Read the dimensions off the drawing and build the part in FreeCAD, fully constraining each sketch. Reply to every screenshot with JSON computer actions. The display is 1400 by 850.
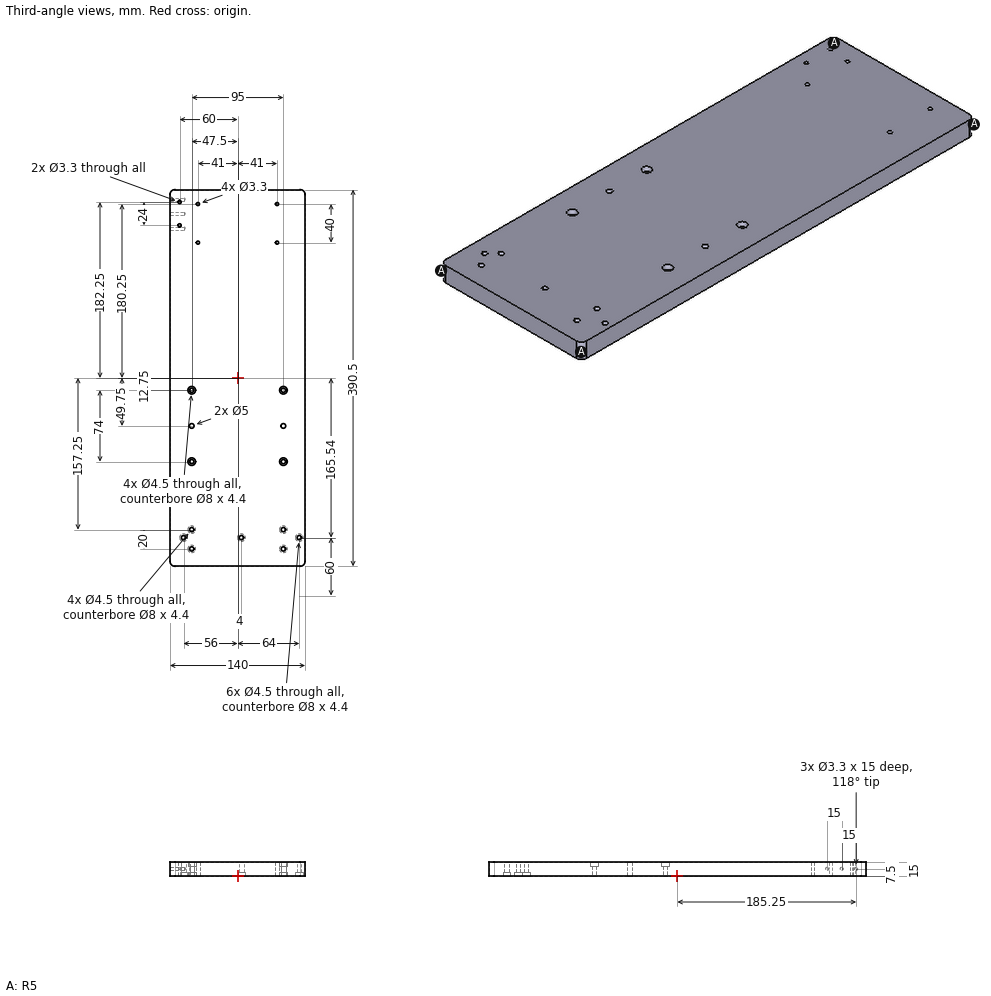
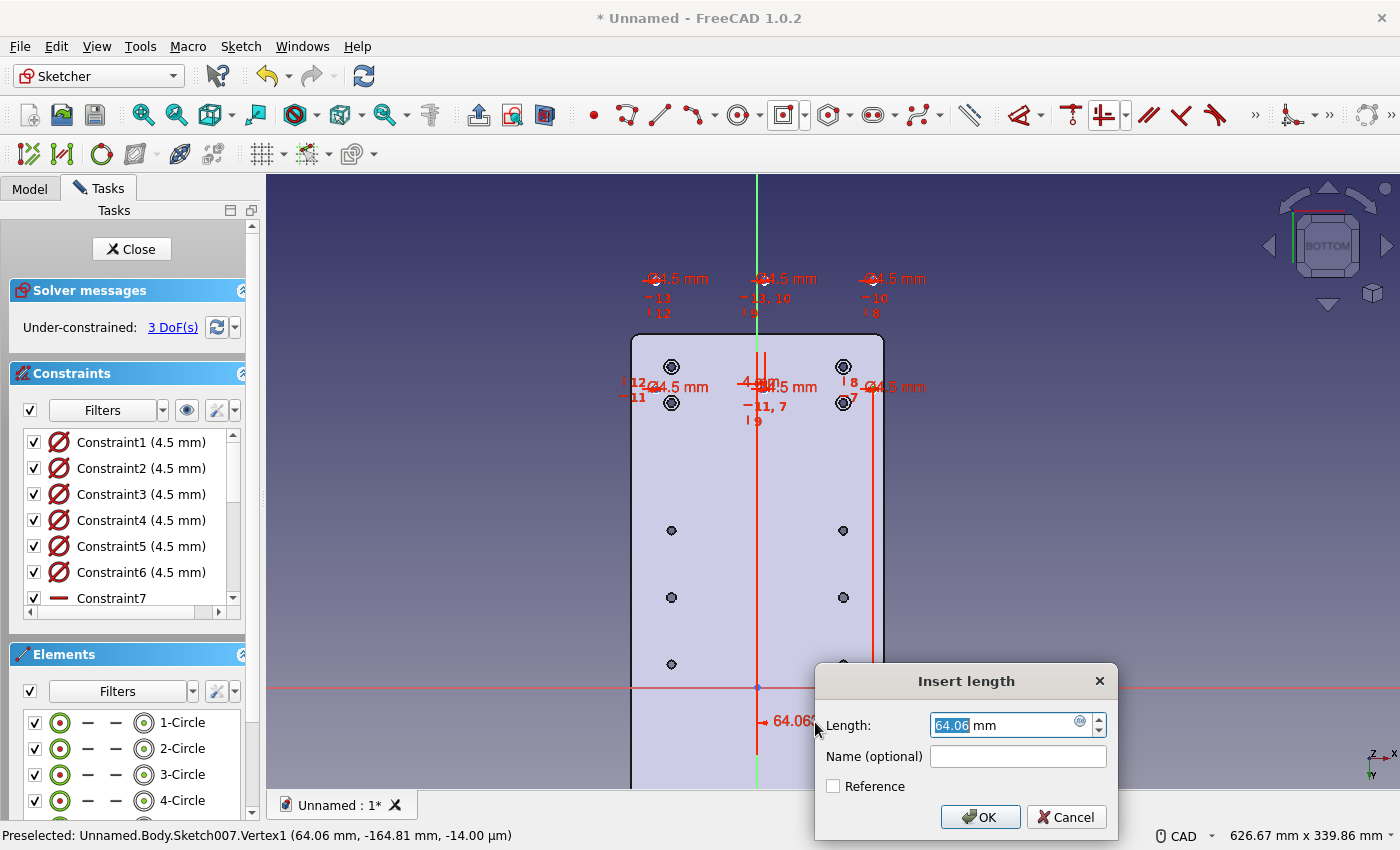
{"action": "type", "text": "64"}
{"action": "key", "text": "Return"}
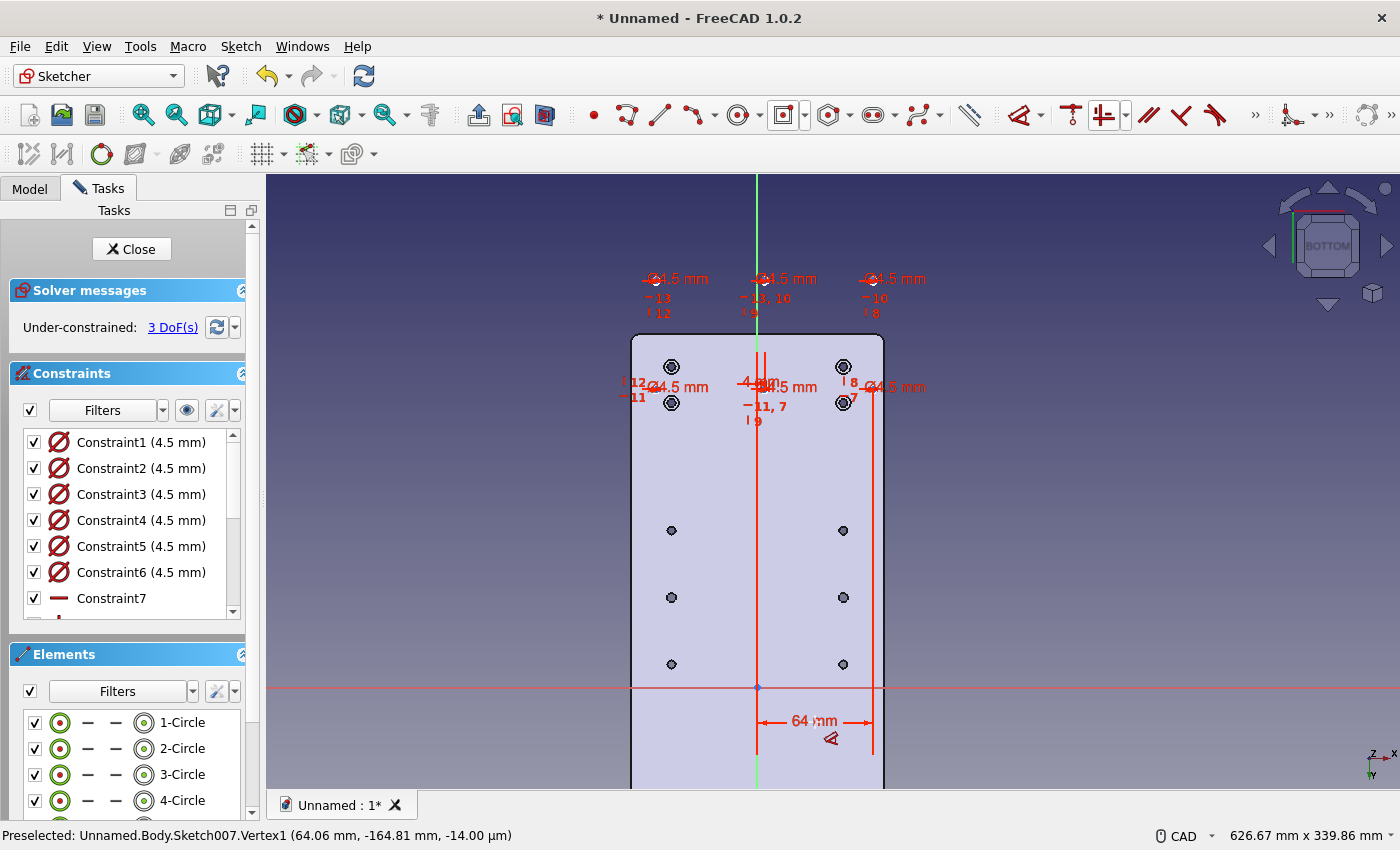
{"action": "left_click", "coordinate": [656, 389]}
{"action": "left_click", "coordinate": [707, 722]}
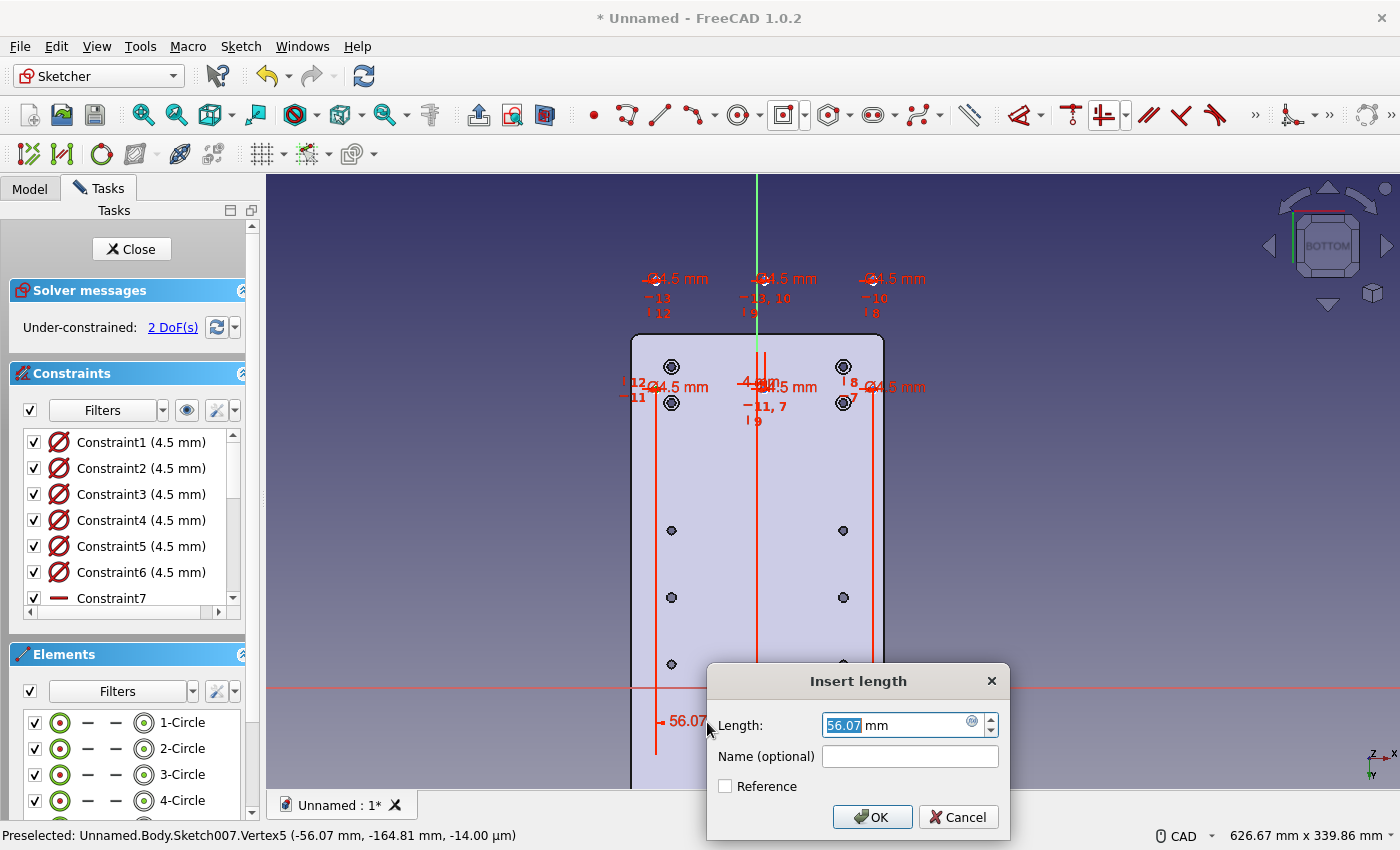
{"action": "type", "text": "56"}
{"action": "key", "text": "Return"}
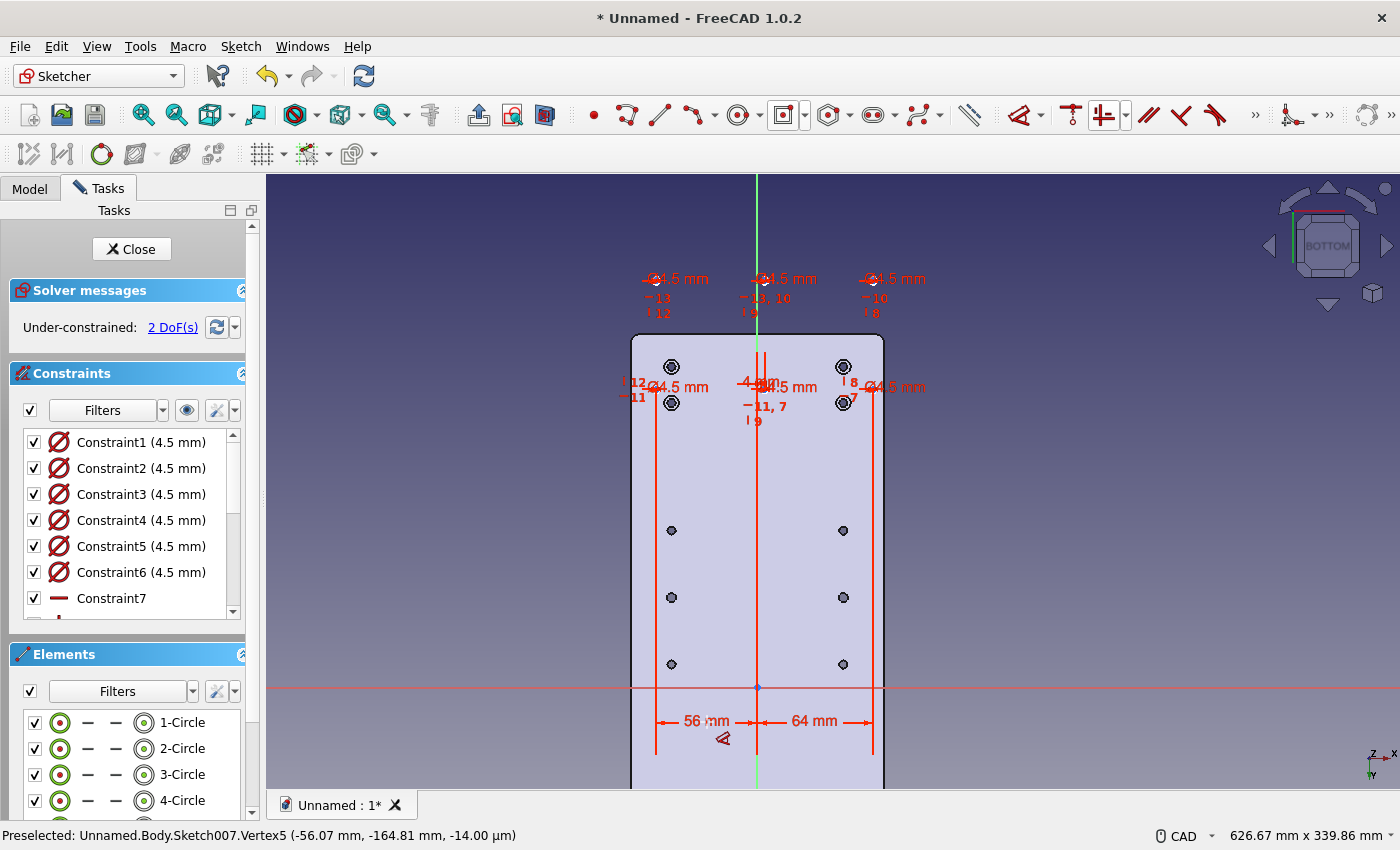
{"action": "left_click", "coordinate": [873, 389]}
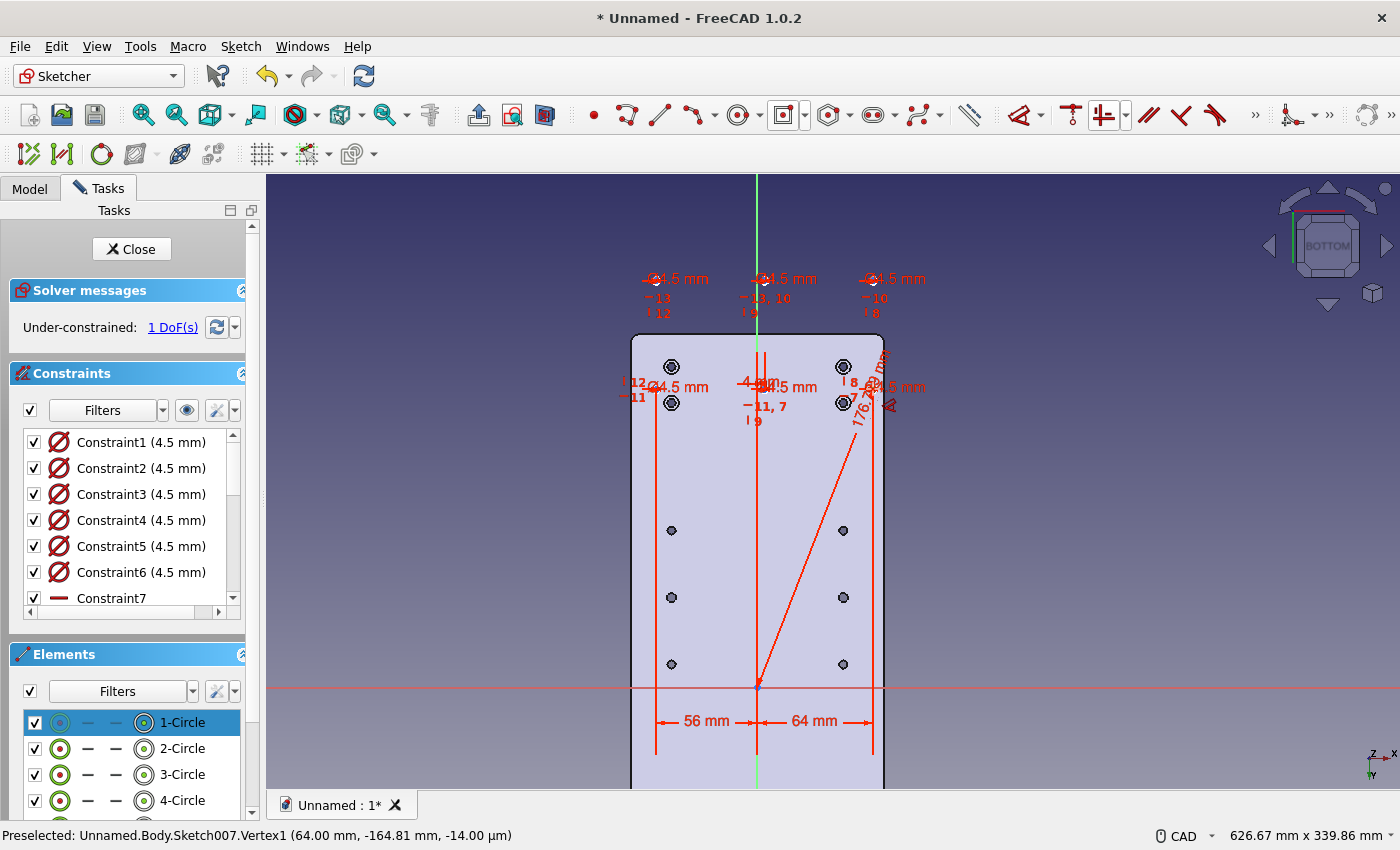
{"action": "left_click", "coordinate": [873, 281]}
{"action": "left_click", "coordinate": [907, 335]}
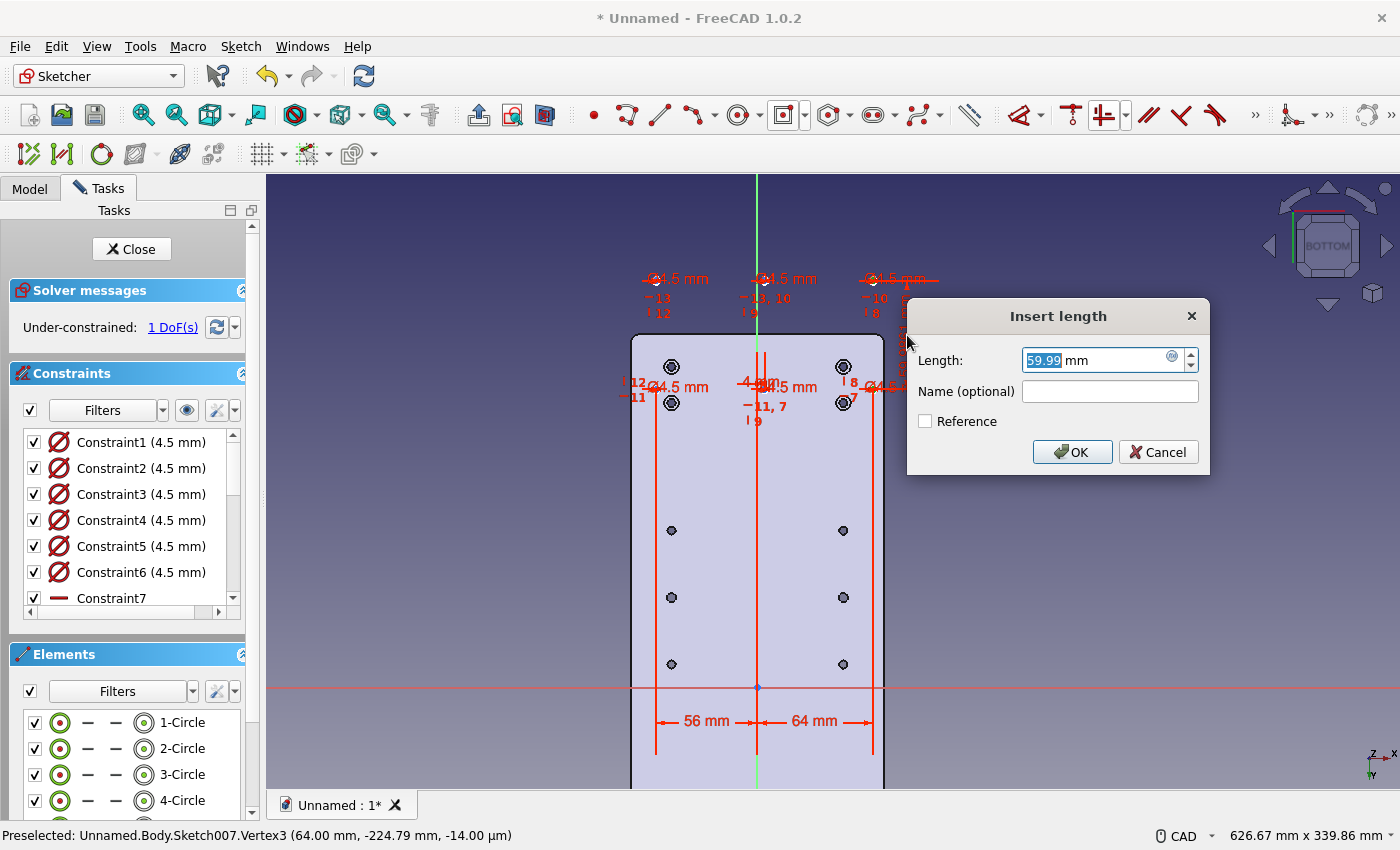
{"action": "type", "text": "60"}
{"action": "key", "text": "Return"}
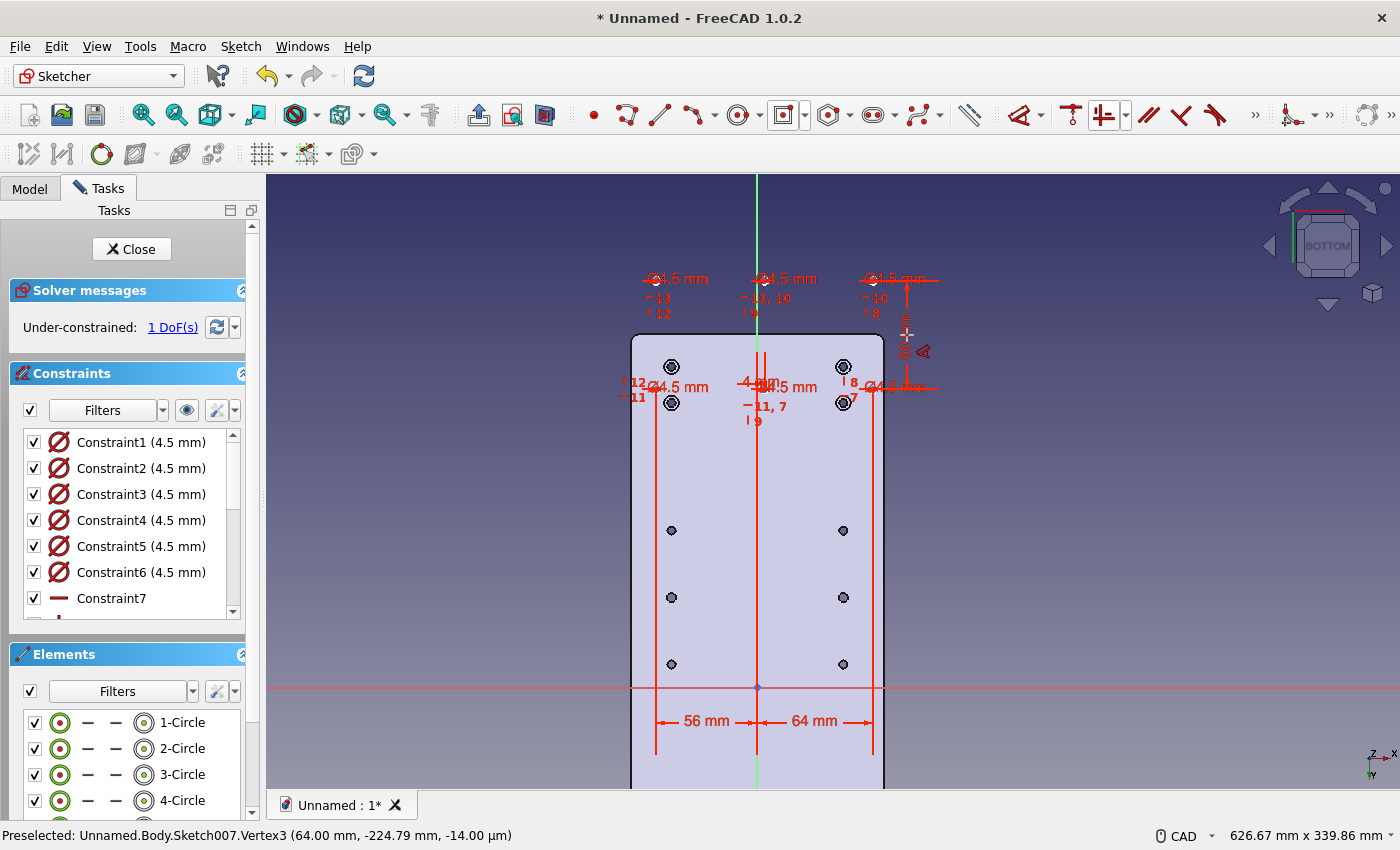
{"action": "left_click", "coordinate": [873, 389]}
{"action": "left_click", "coordinate": [907, 538]}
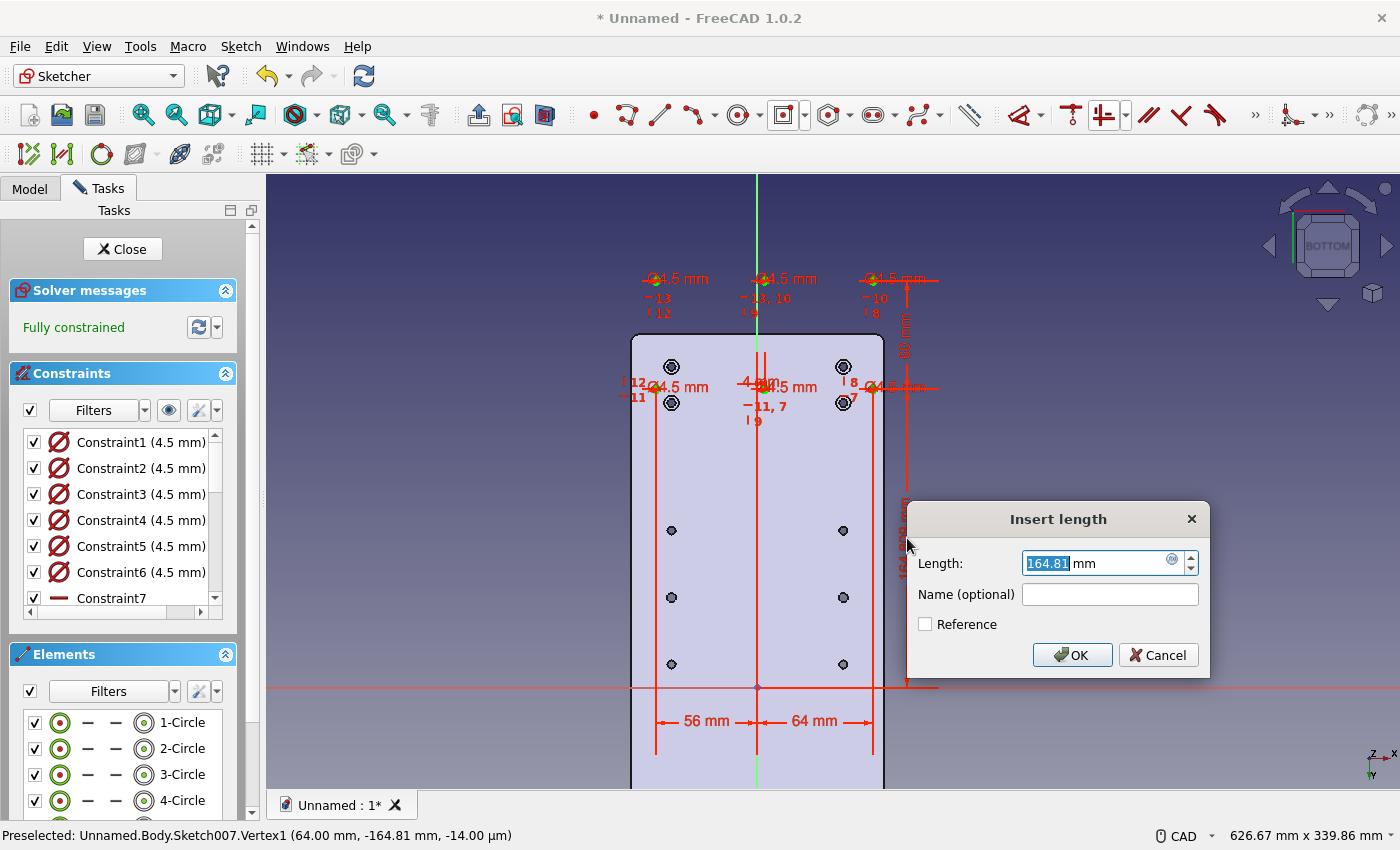
{"action": "type", "text": "165.54"}
{"action": "key", "text": "Return"}
{"action": "key", "text": "Escape"}